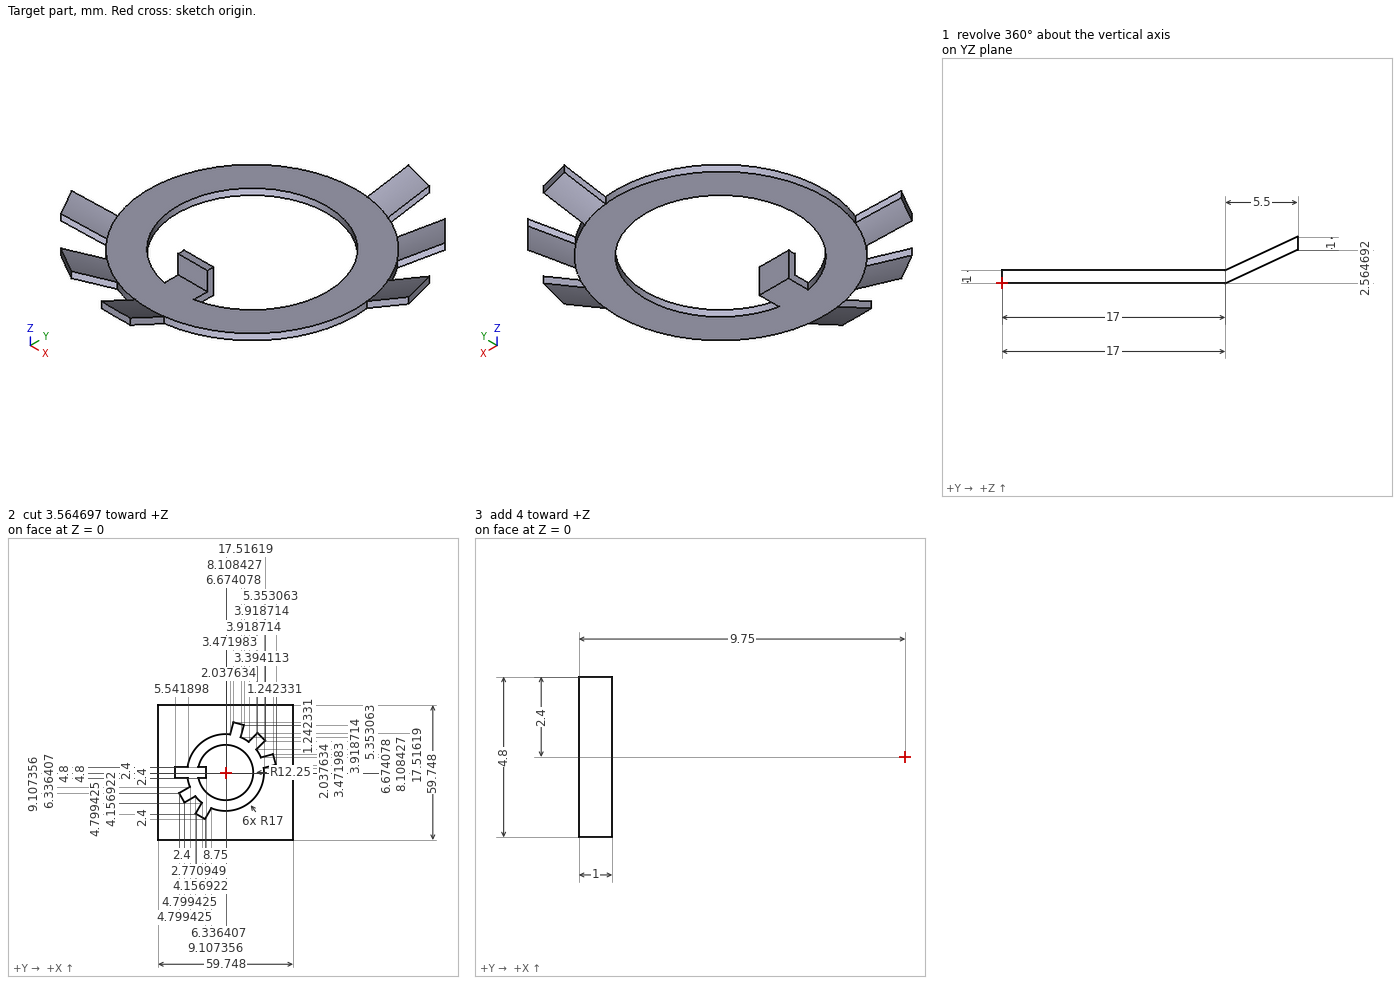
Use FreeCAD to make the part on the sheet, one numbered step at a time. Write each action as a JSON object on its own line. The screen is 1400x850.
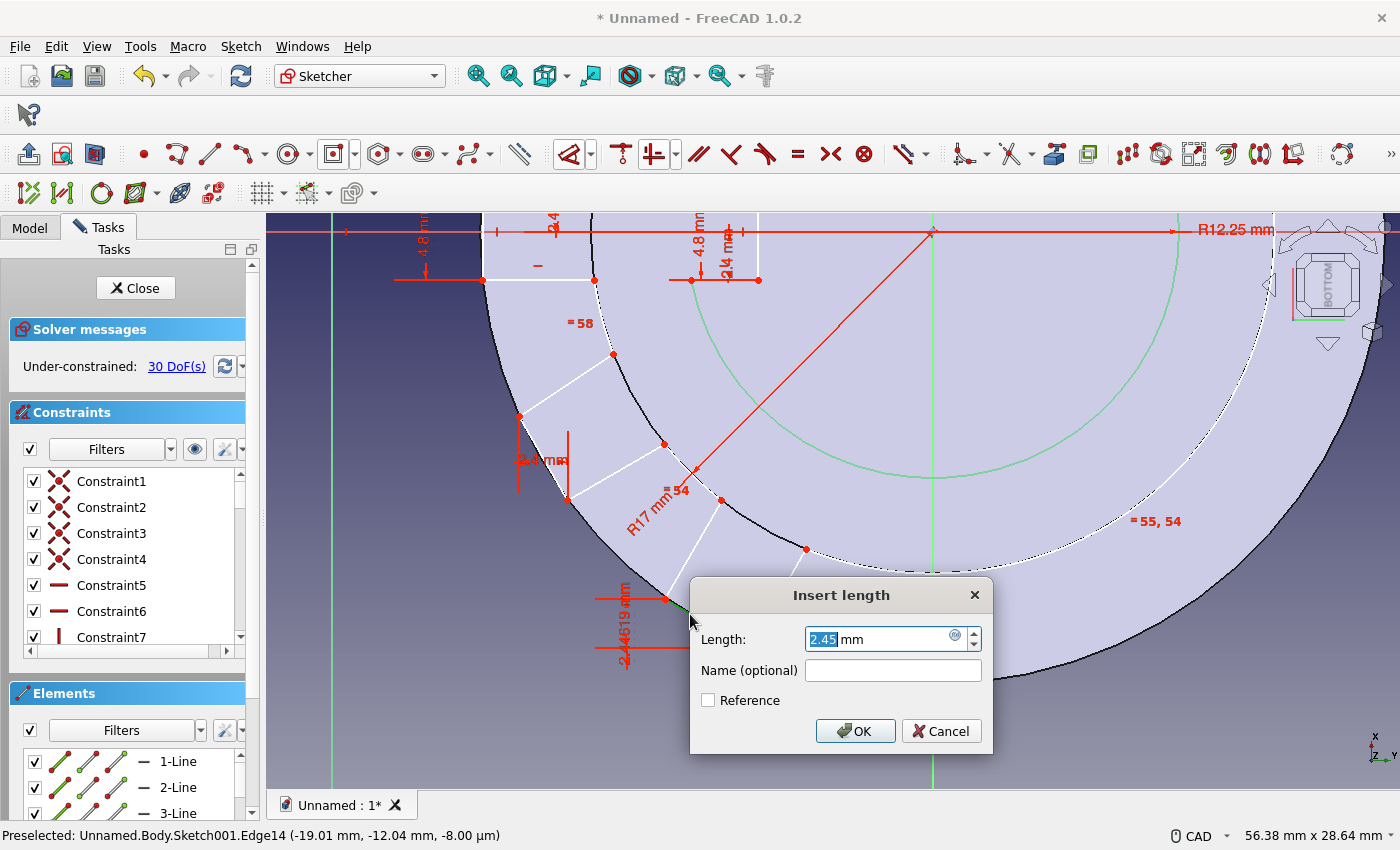
{"action": "type", "text": "2.4"}
{"action": "key", "text": "Return"}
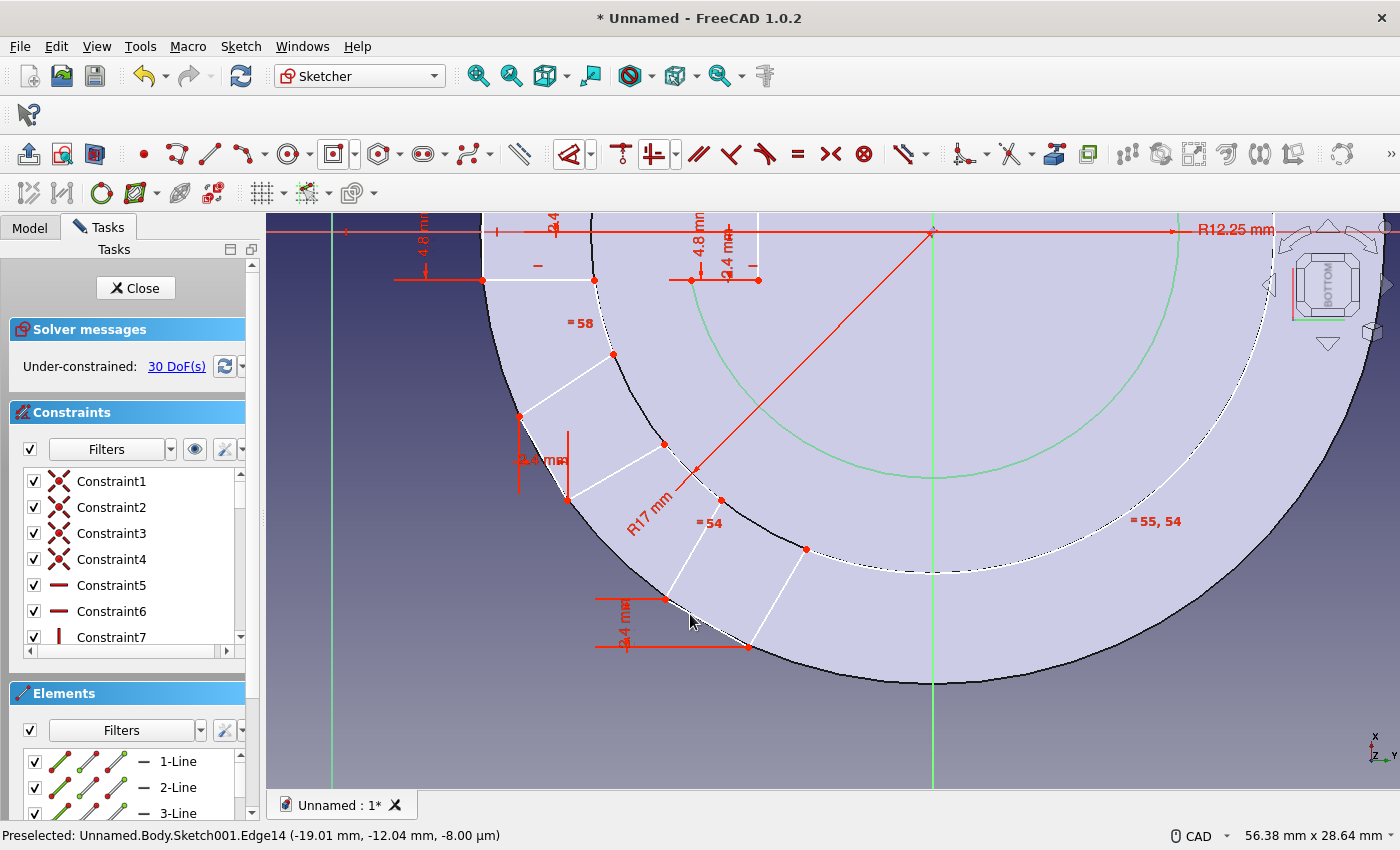
{"action": "left_click", "coordinate": [758, 280]}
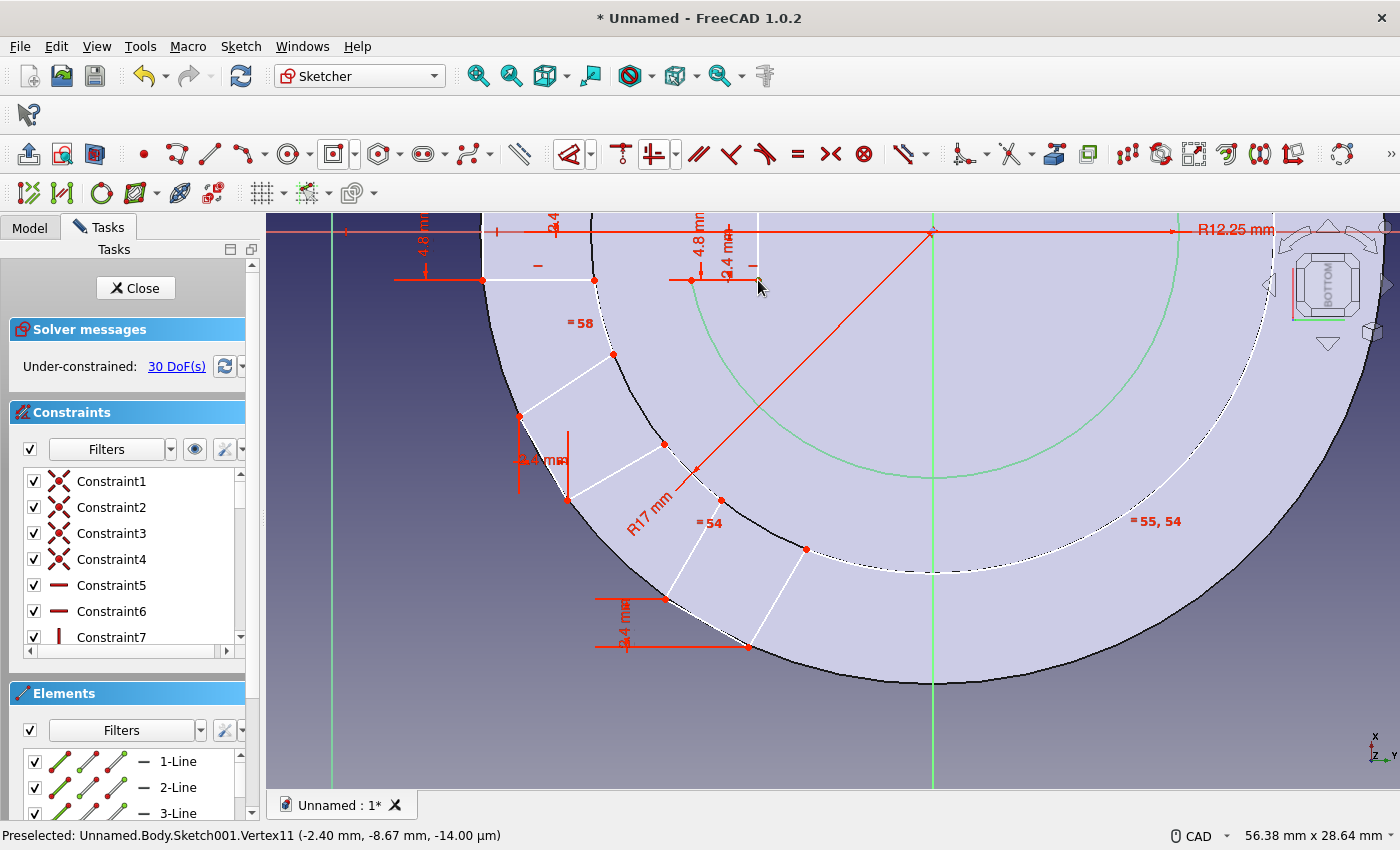
{"action": "left_click", "coordinate": [590, 154]}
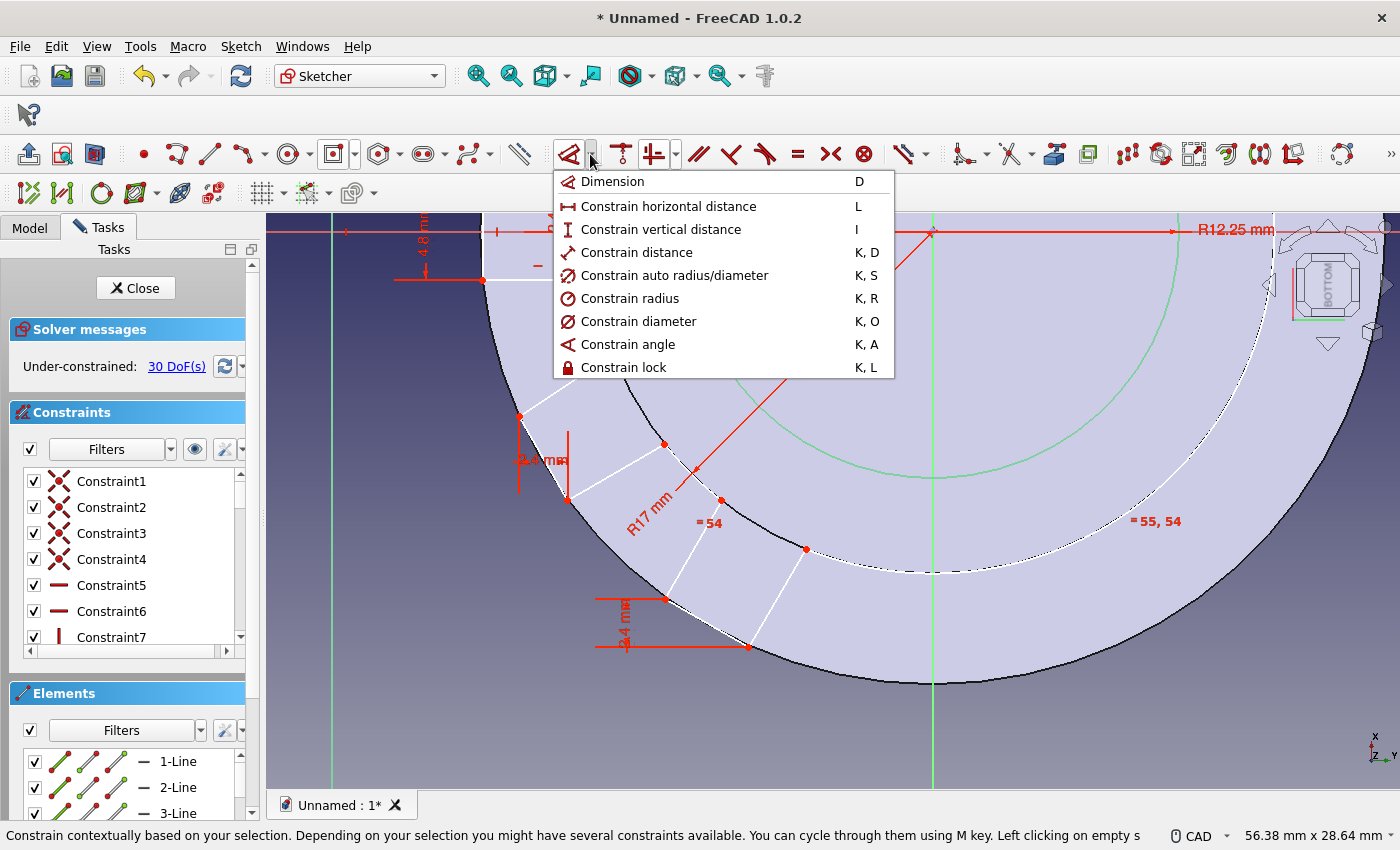
{"action": "left_click", "coordinate": [724, 206]}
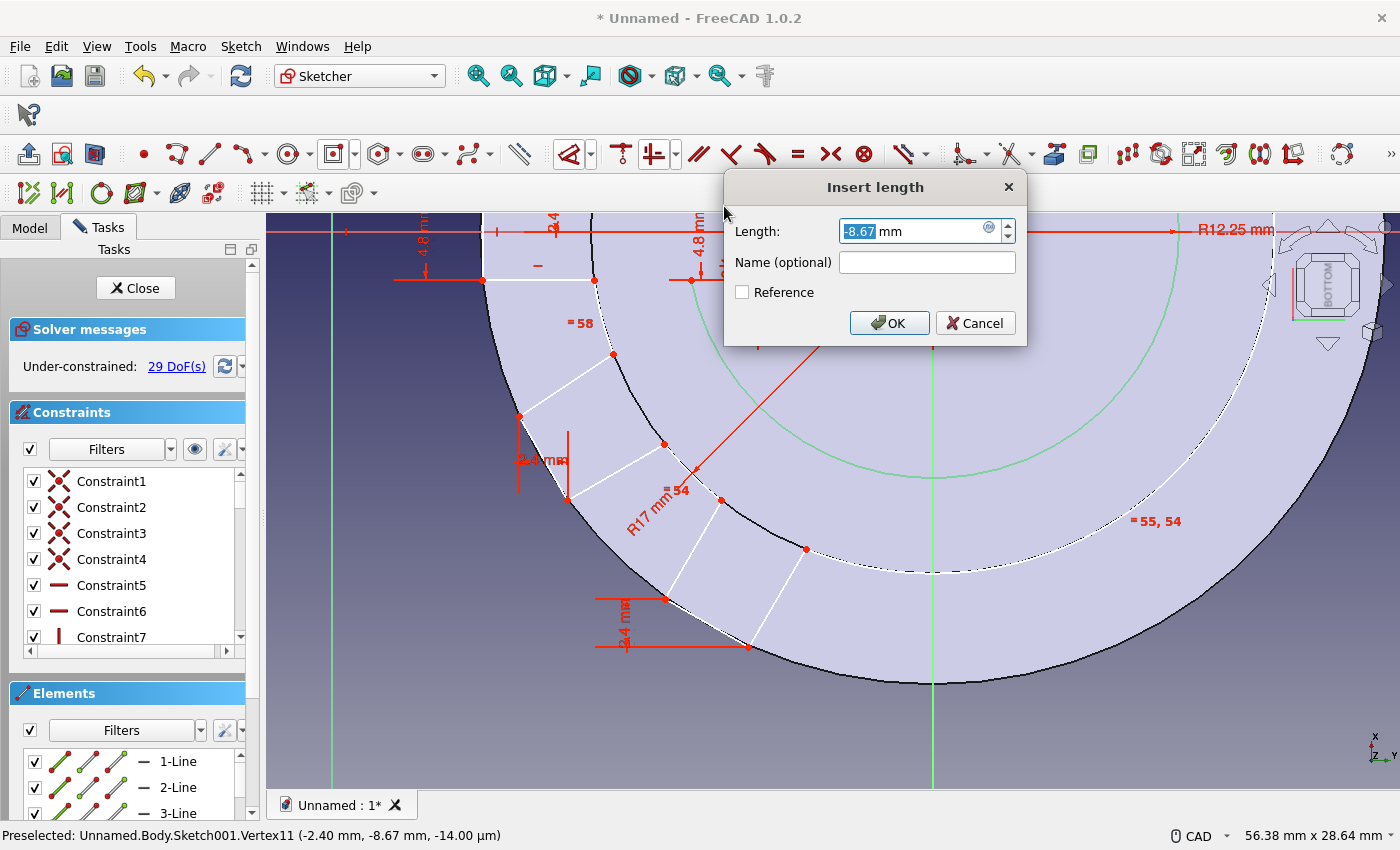
{"action": "type", "text": "-8.75"}
{"action": "key", "text": "Return"}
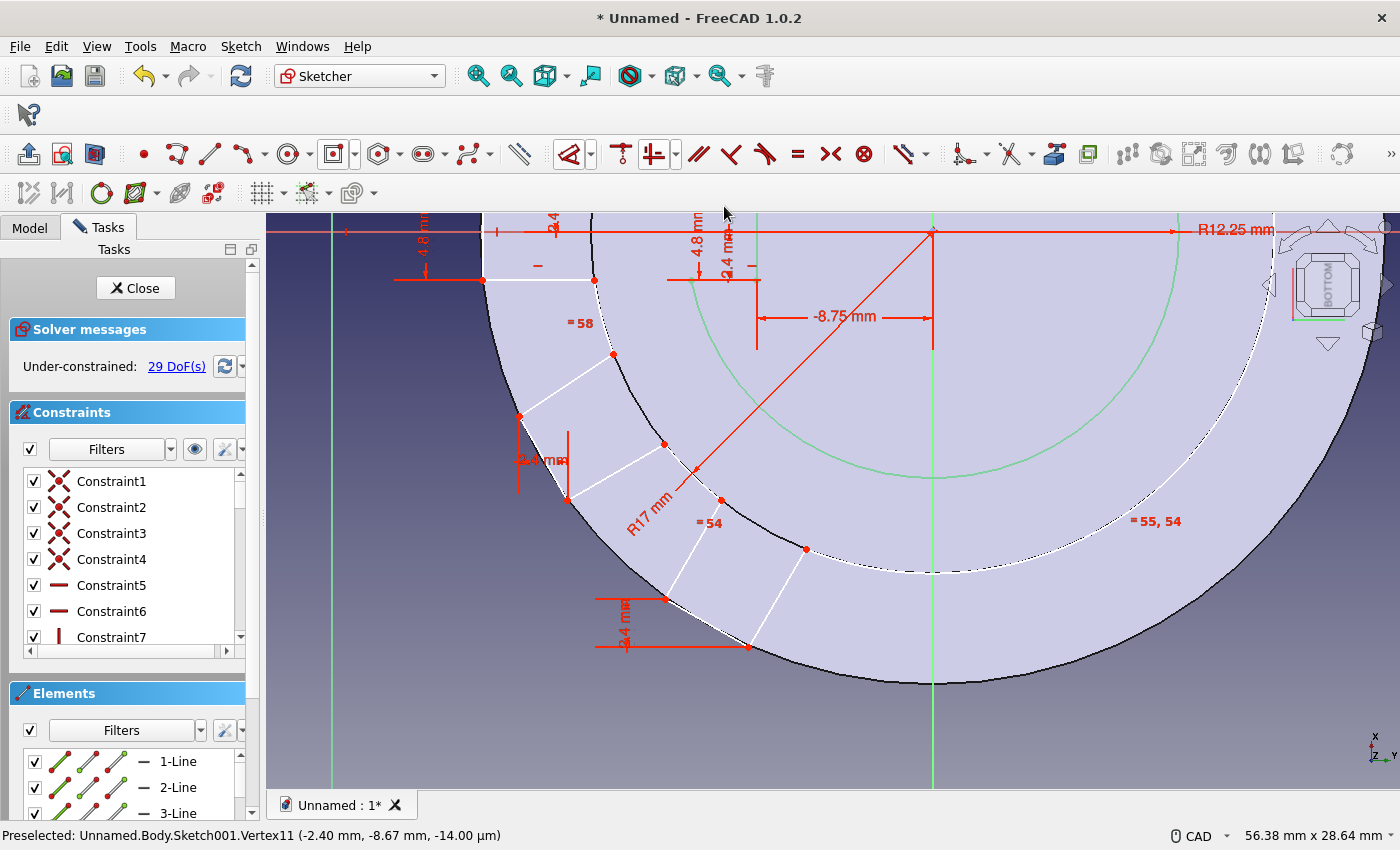
{"action": "scroll", "coordinate": [692, 617], "scroll_direction": "down", "scroll_amount": 6}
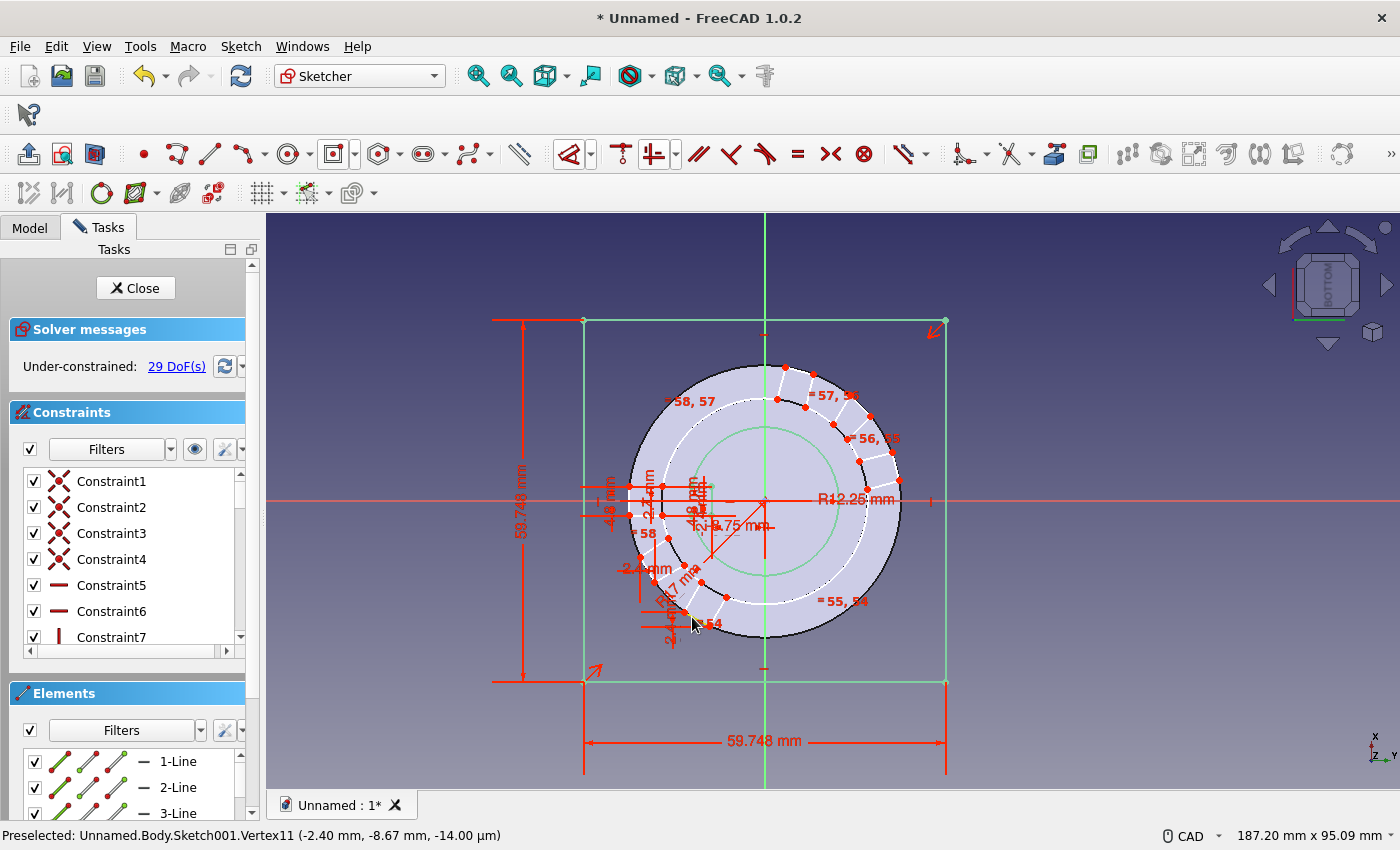
{"action": "scroll", "coordinate": [653, 487], "scroll_direction": "up", "scroll_amount": 2}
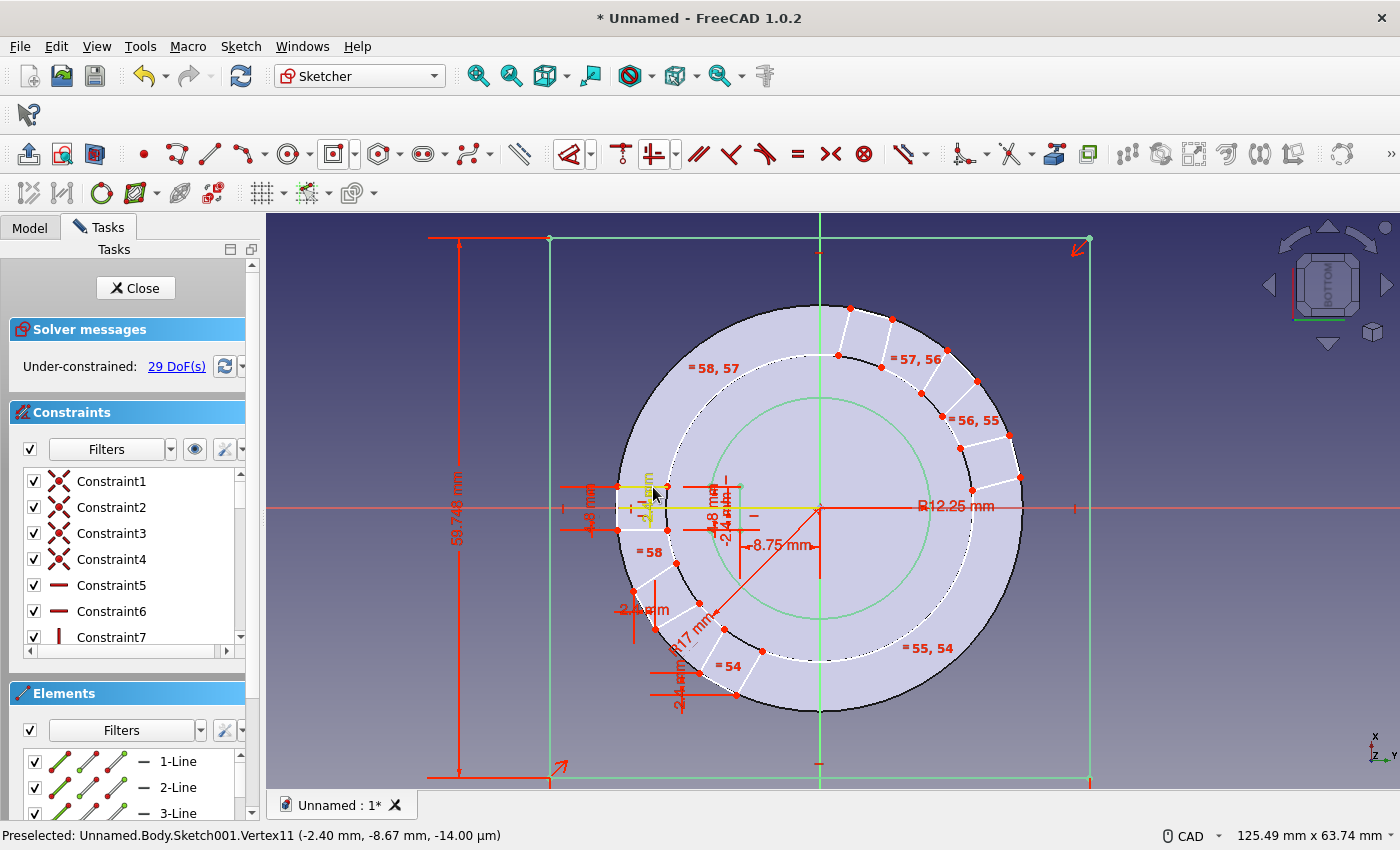
{"action": "left_click", "coordinate": [632, 487]}